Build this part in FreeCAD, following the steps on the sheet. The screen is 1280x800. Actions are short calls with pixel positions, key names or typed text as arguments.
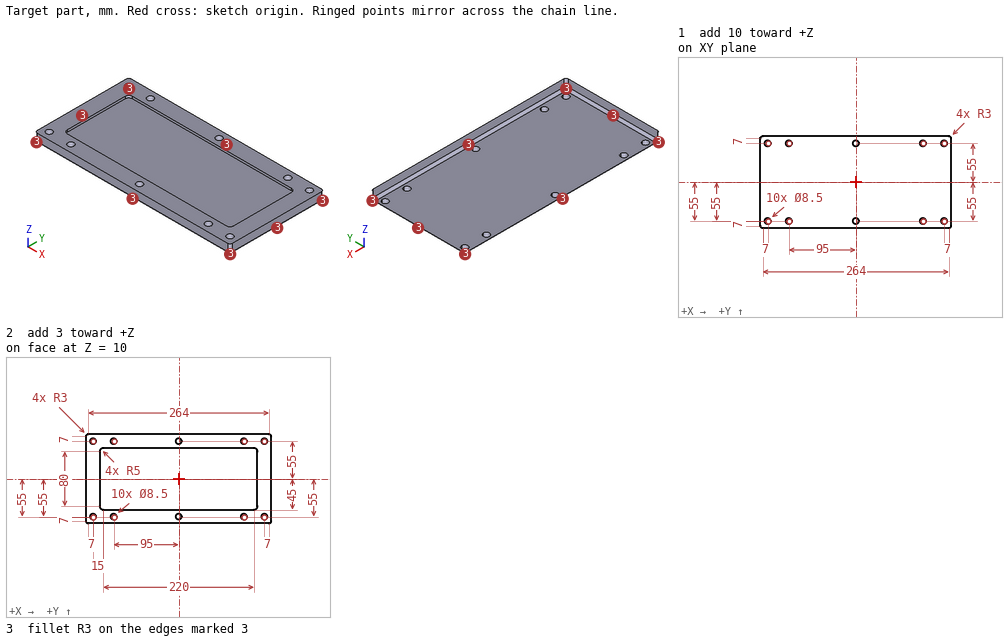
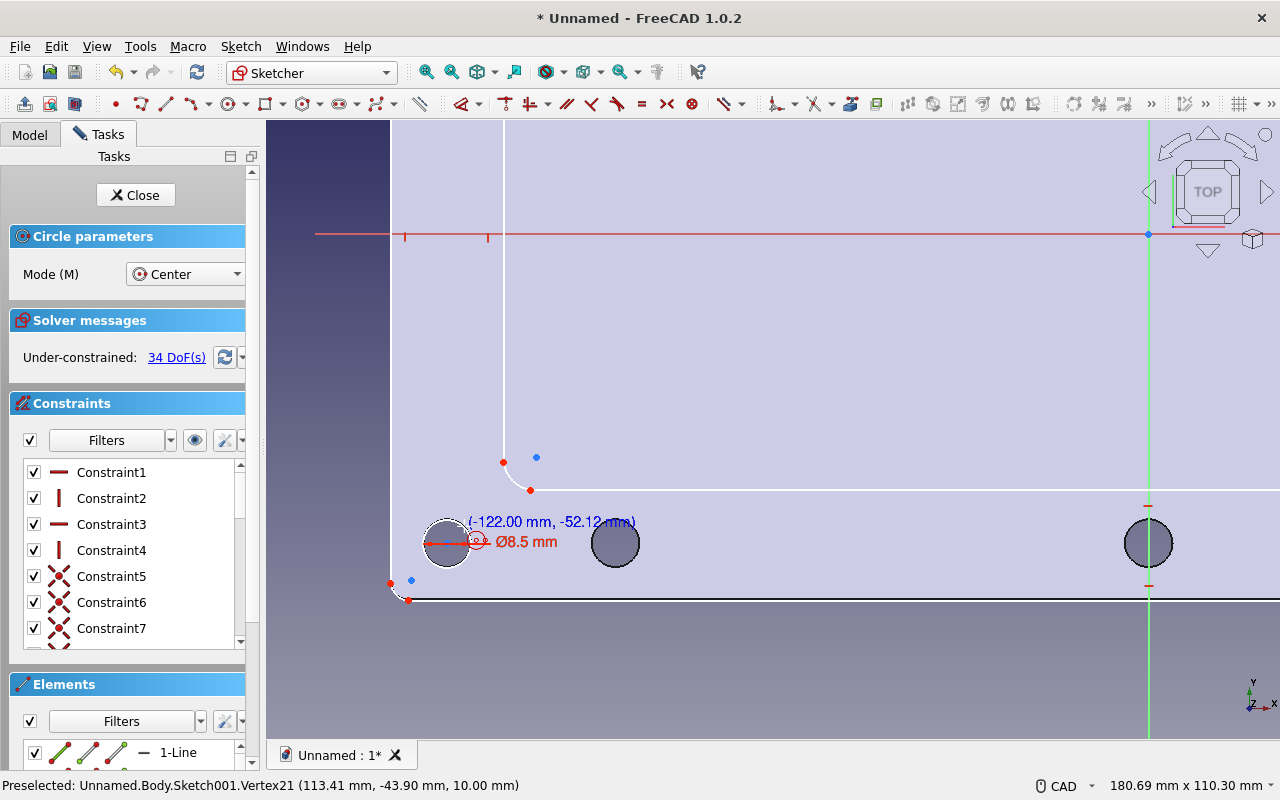
click(616, 543)
move(632, 526)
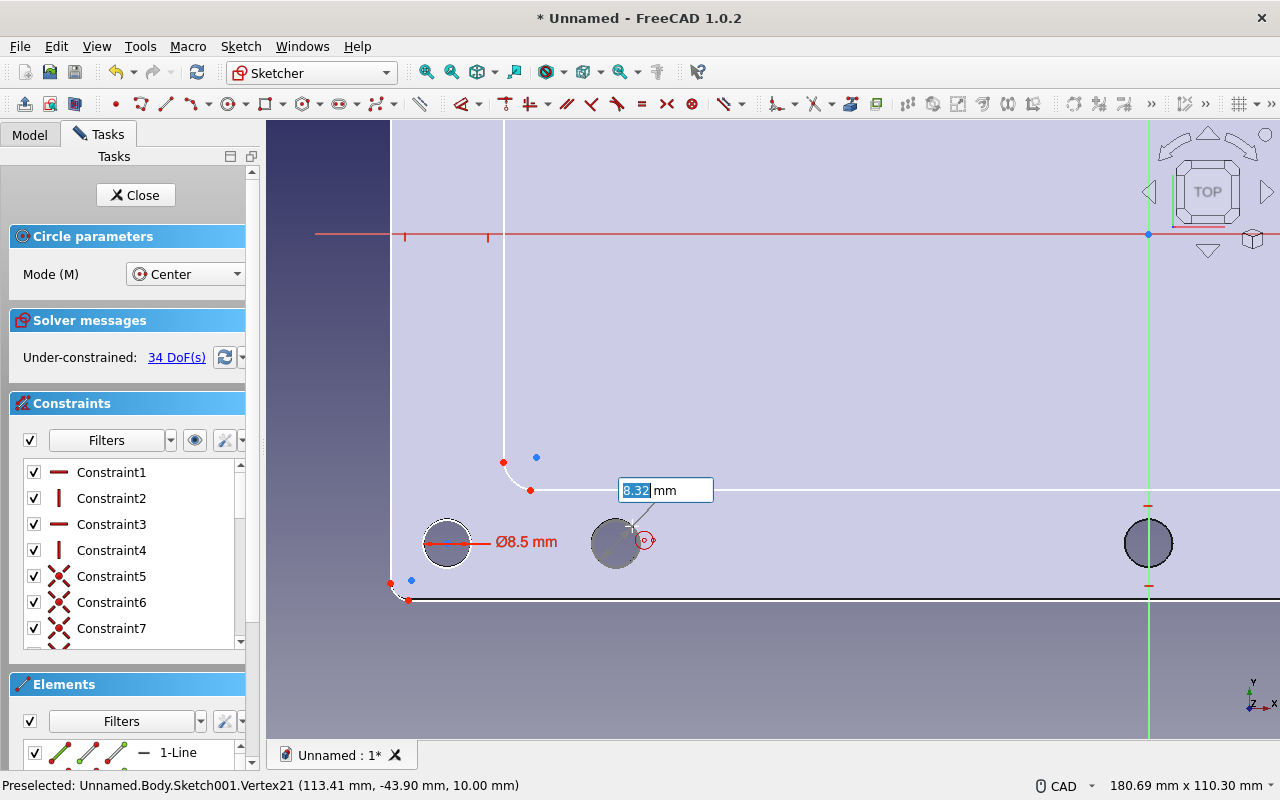
text(8.5)
key(Return)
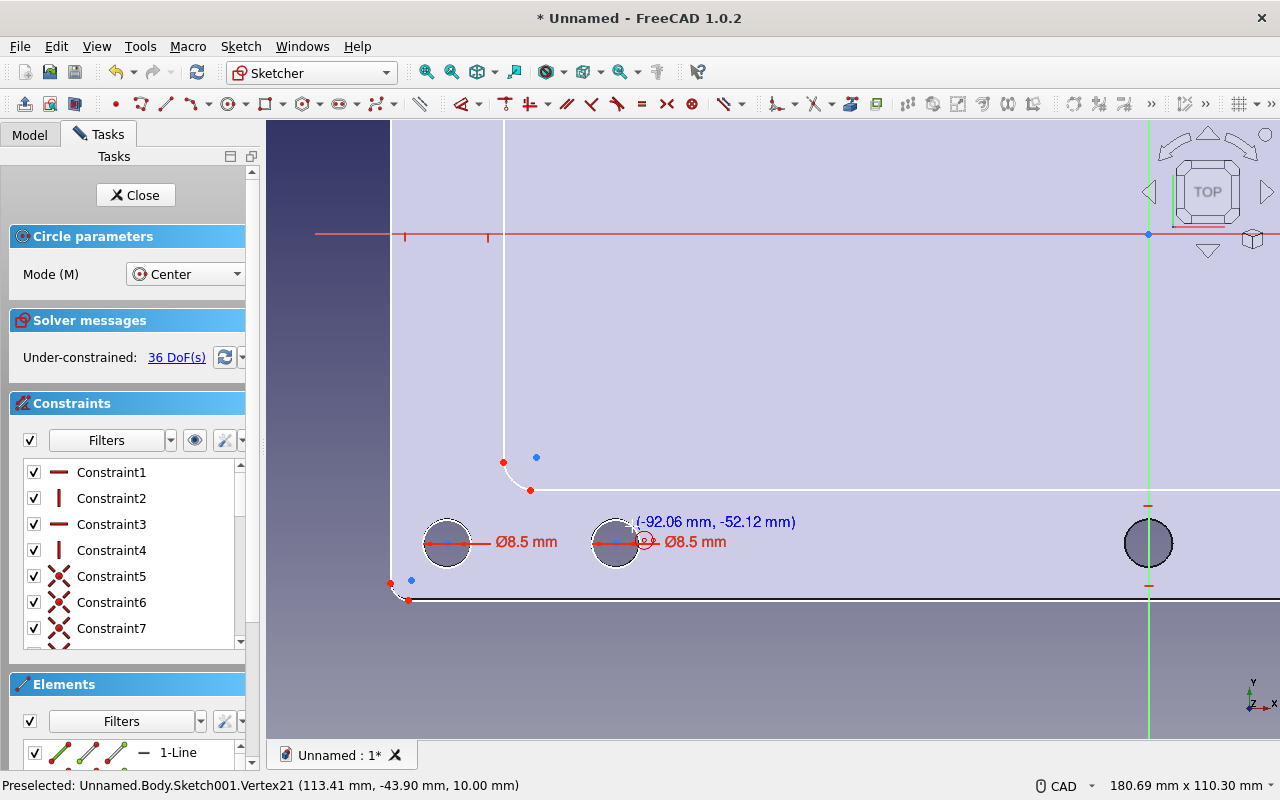
scroll(446, 543, down, 5)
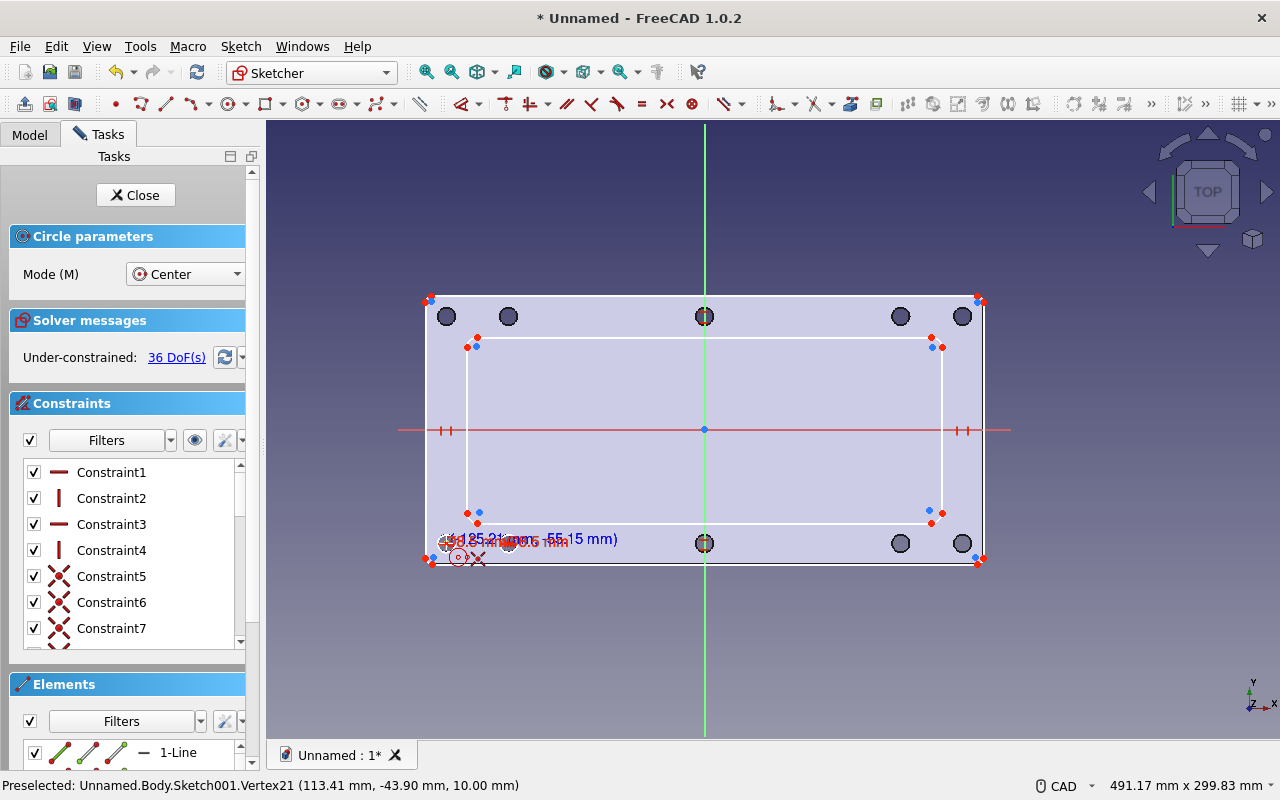
scroll(705, 543, up, 5)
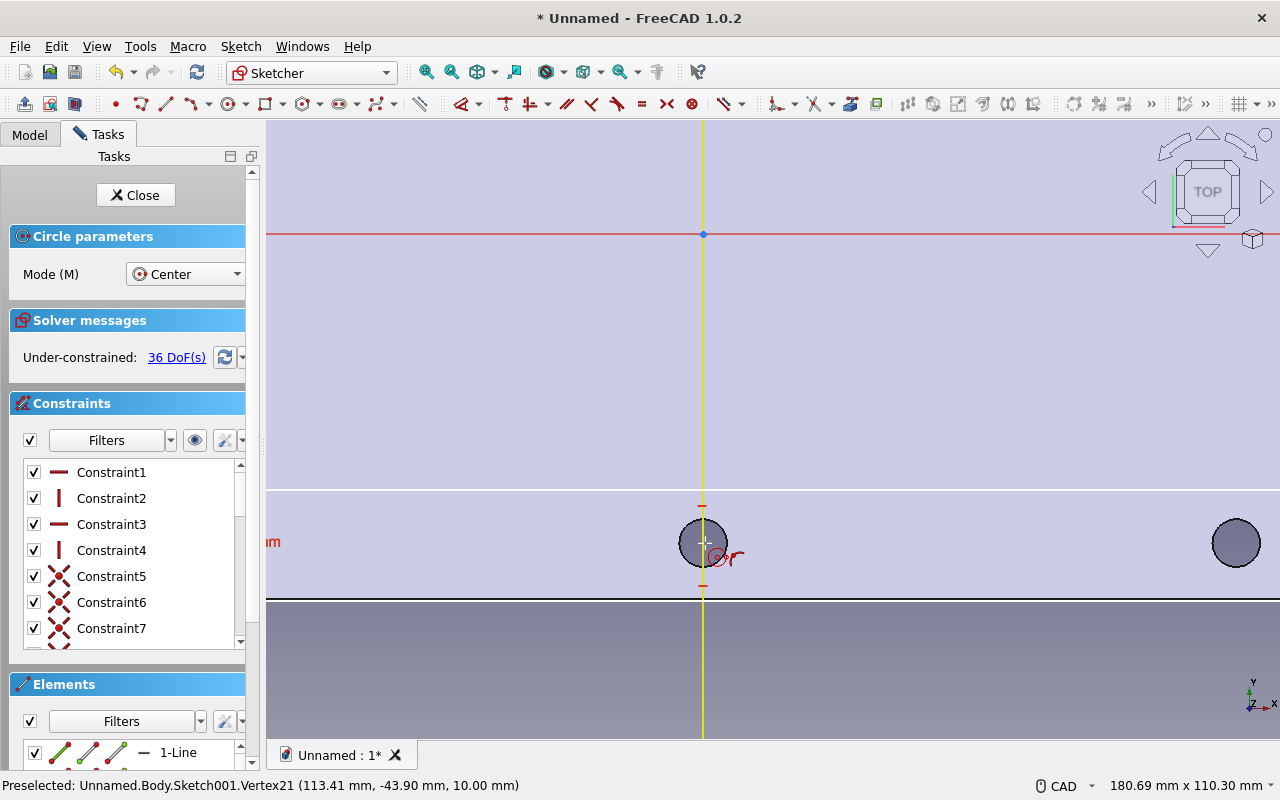
click(703, 543)
move(720, 526)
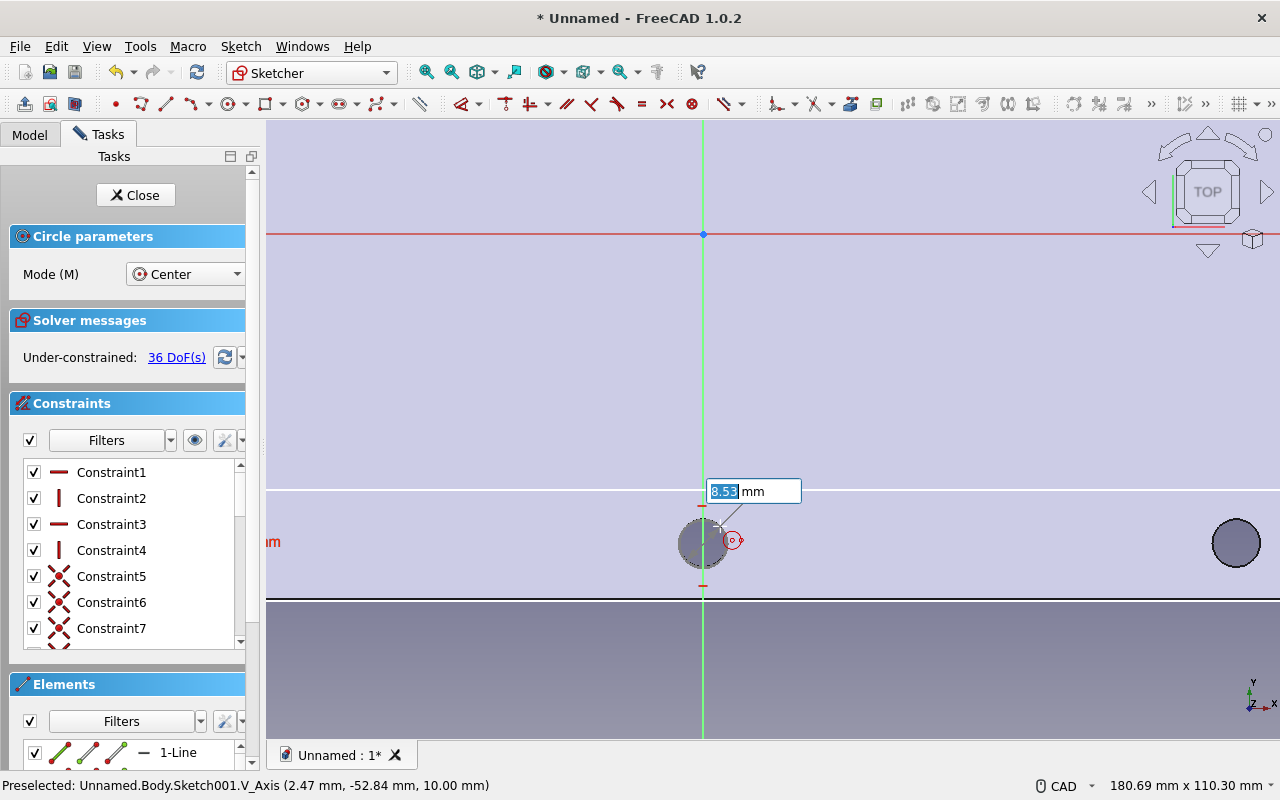
text(8.5)
key(Return)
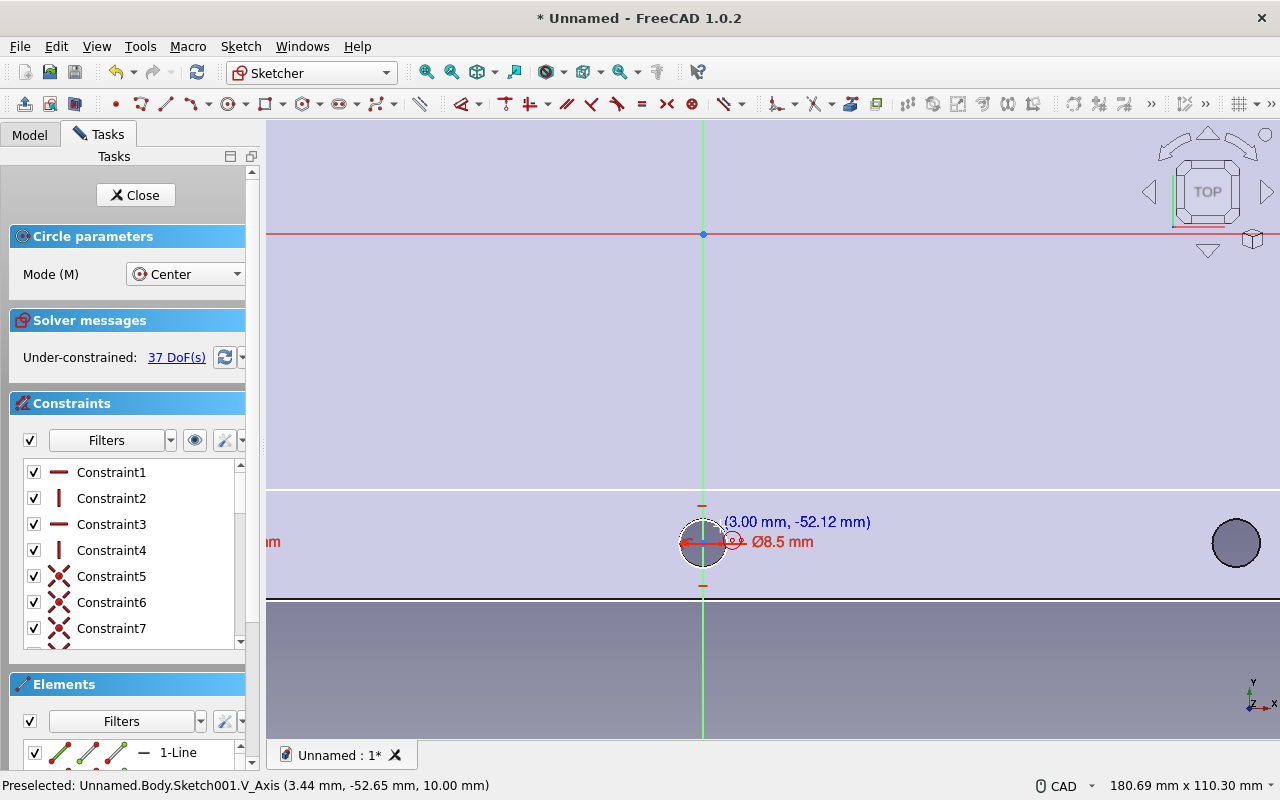
scroll(705, 543, down, 5)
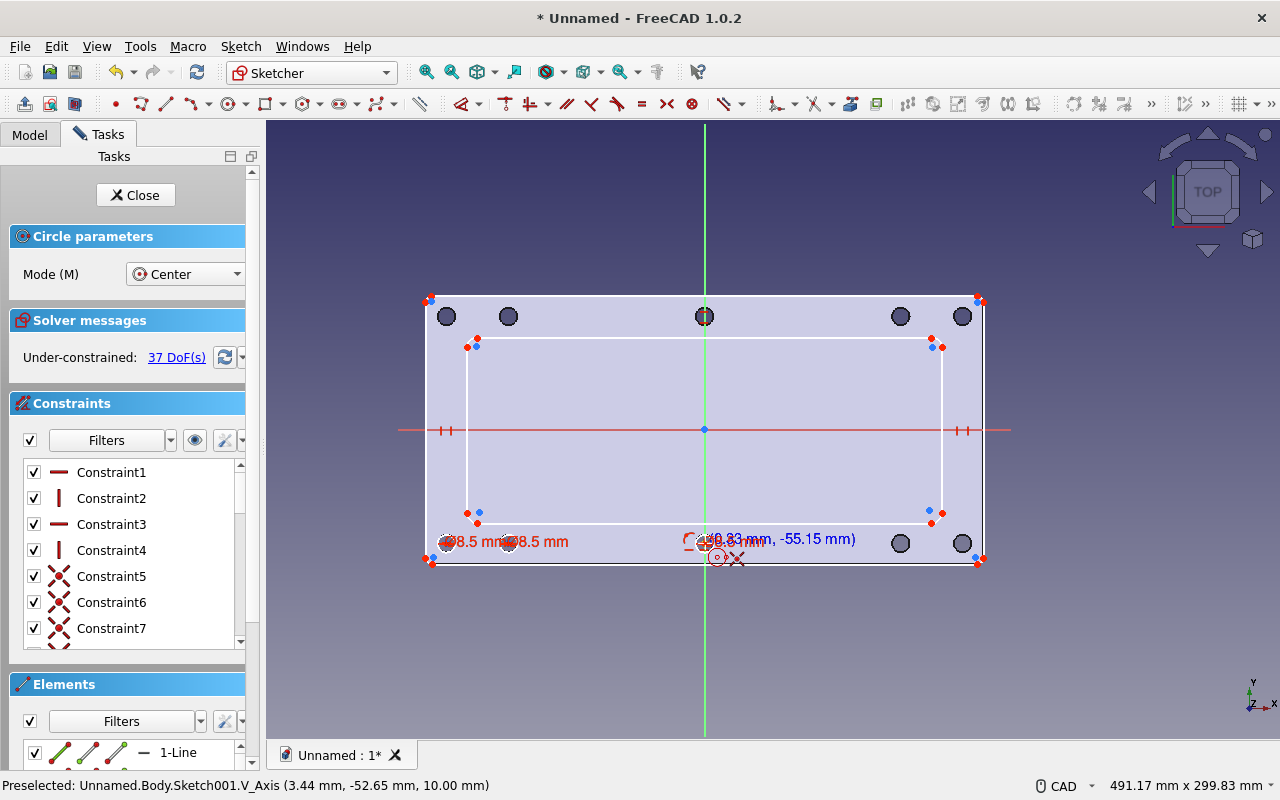
scroll(901, 543, up, 5)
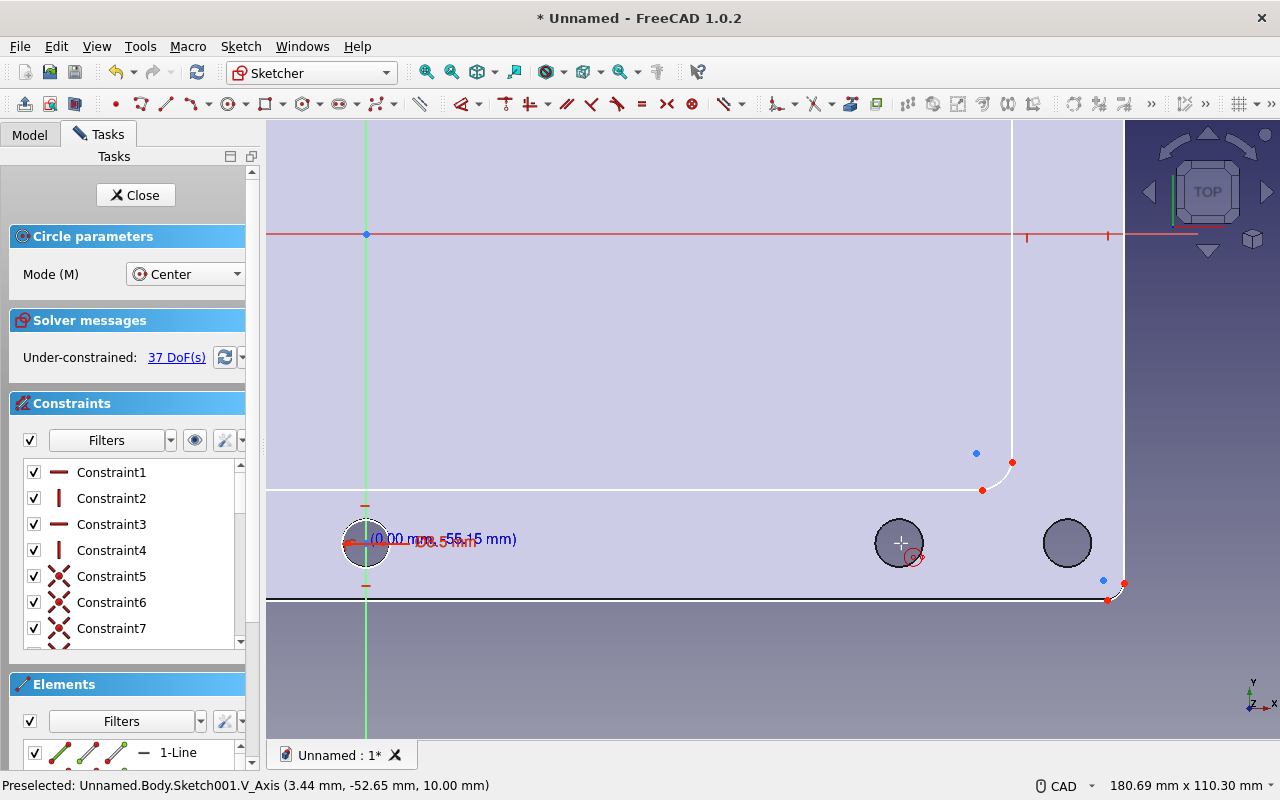
click(899, 543)
move(916, 526)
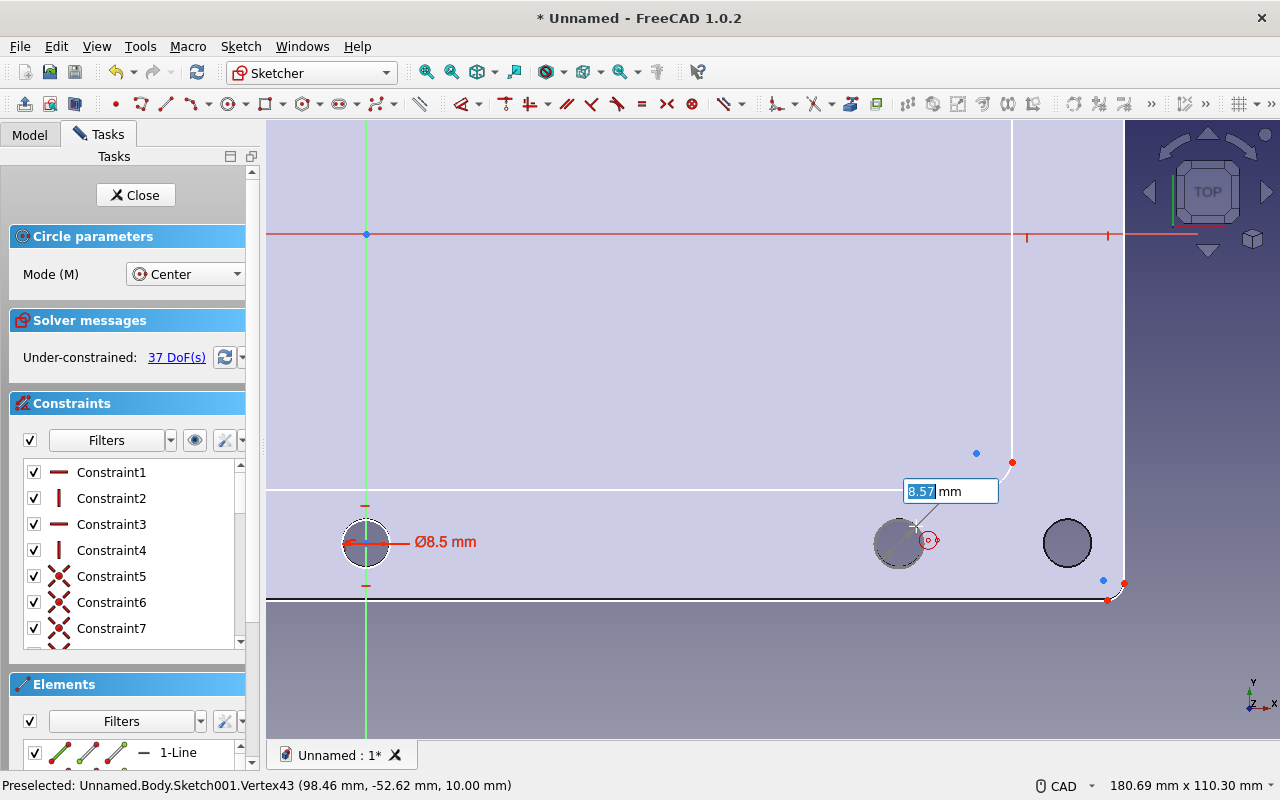
text(8.5)
key(Return)